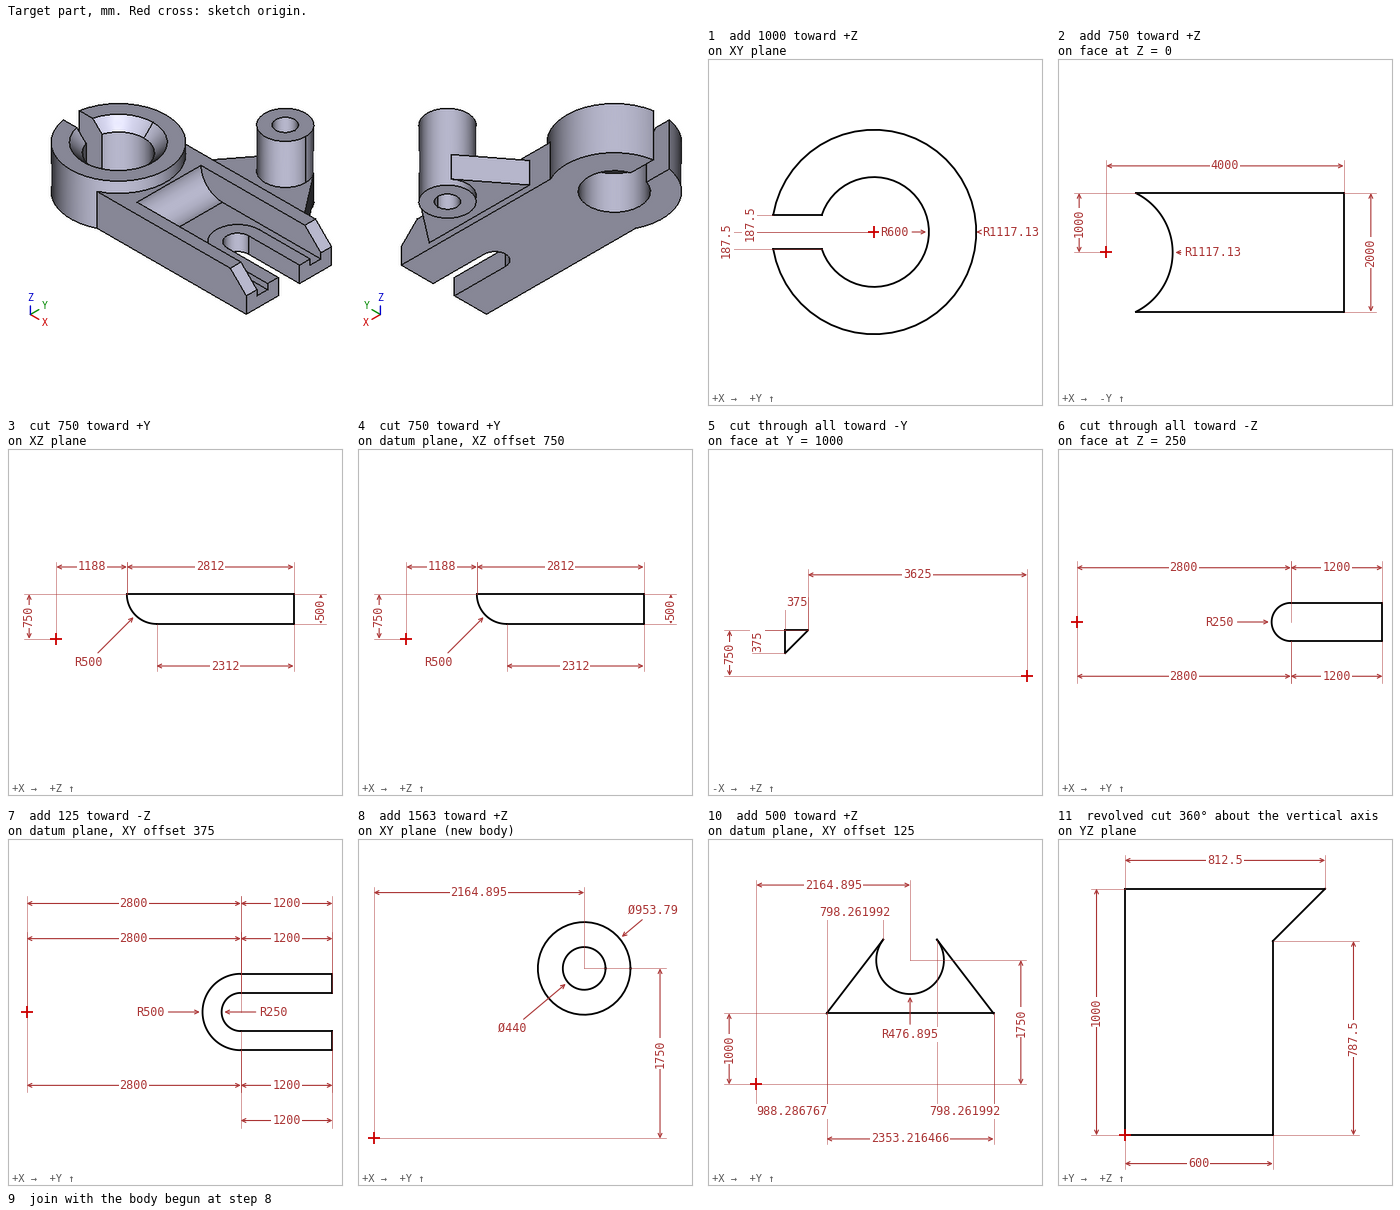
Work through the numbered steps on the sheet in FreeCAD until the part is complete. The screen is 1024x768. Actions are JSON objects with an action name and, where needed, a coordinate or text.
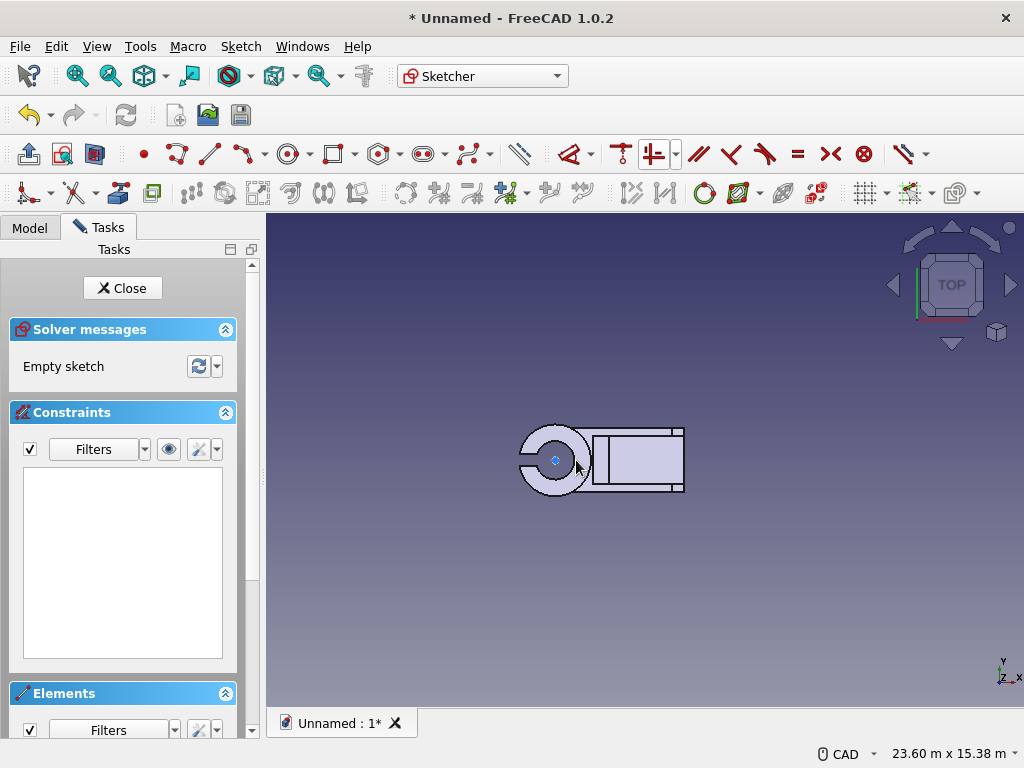
{"action": "scroll", "coordinate": [671, 460], "scroll_direction": "up", "scroll_amount": 11}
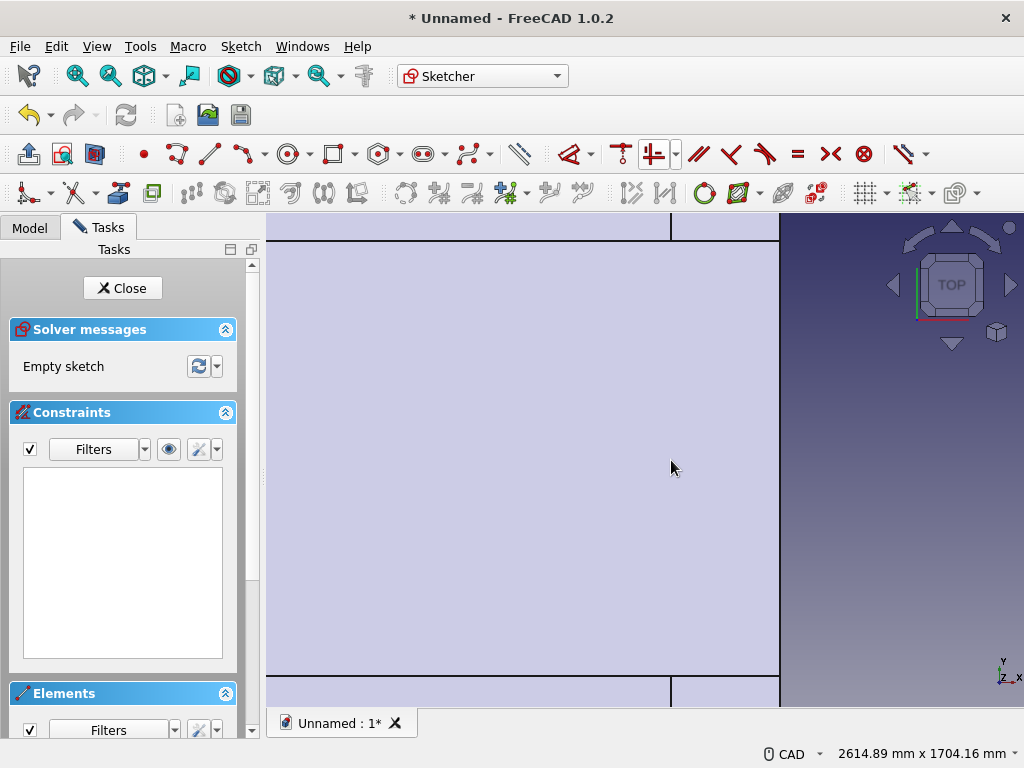
{"action": "key", "text": "g m"}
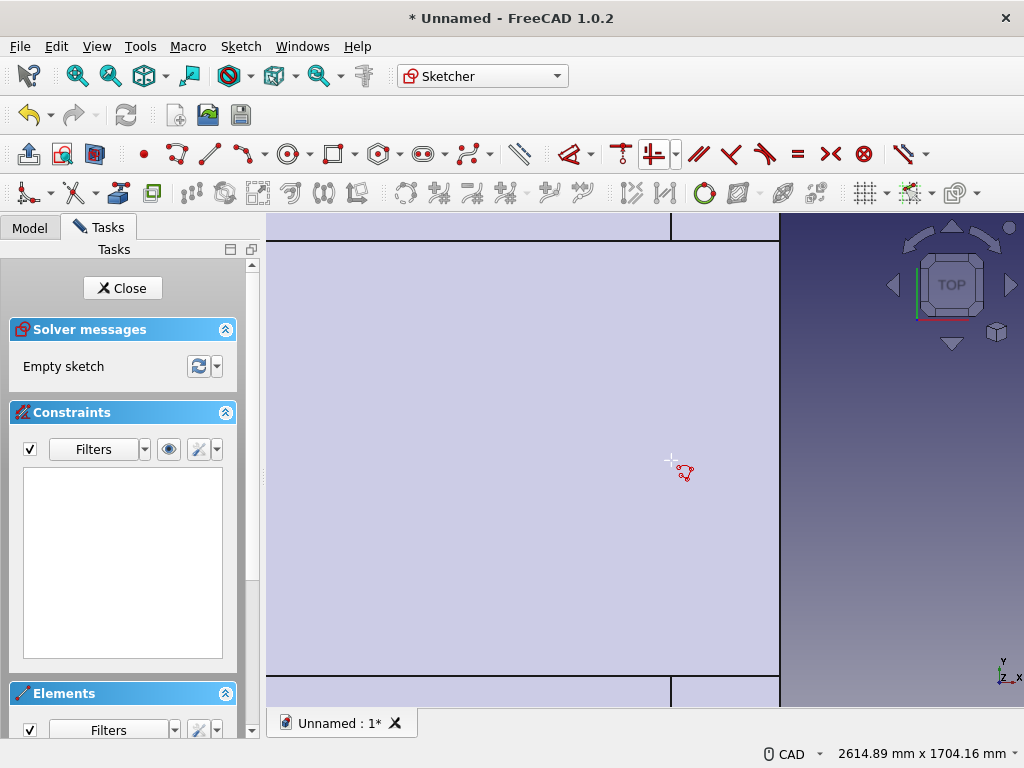
{"action": "left_click", "coordinate": [432, 531]}
{"action": "left_click", "coordinate": [780, 531]}
{"action": "left_click", "coordinate": [780, 386]}
{"action": "left_click", "coordinate": [432, 386]}
{"action": "right_click", "coordinate": [432, 386]}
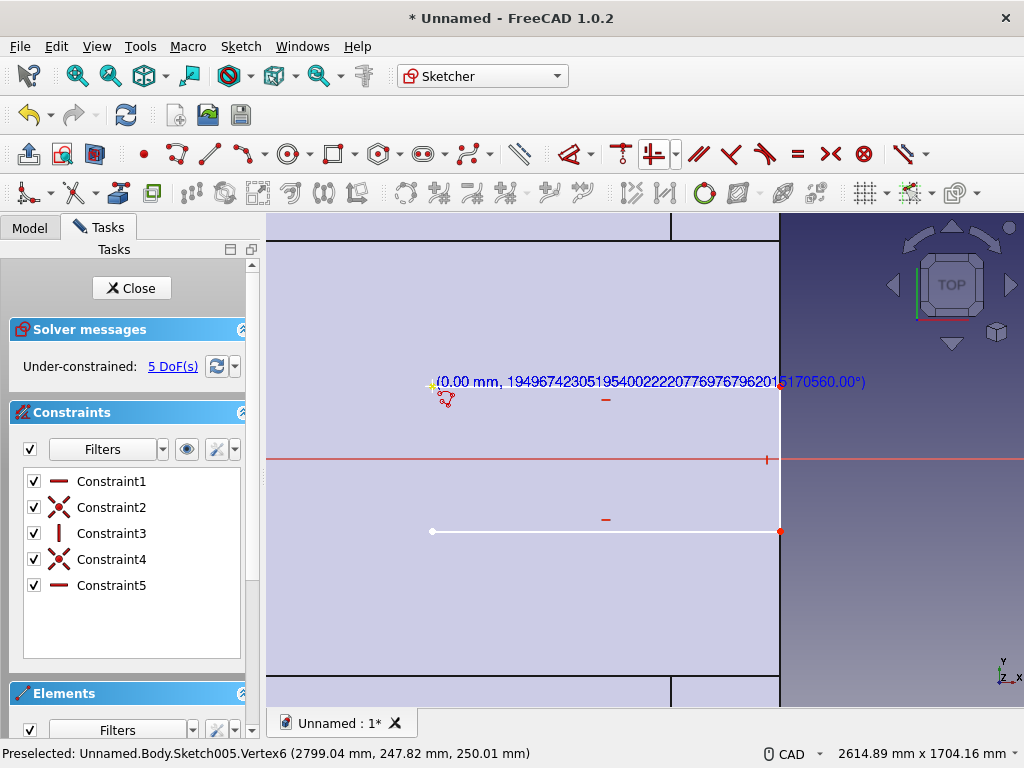
{"action": "key", "text": "g 3 a"}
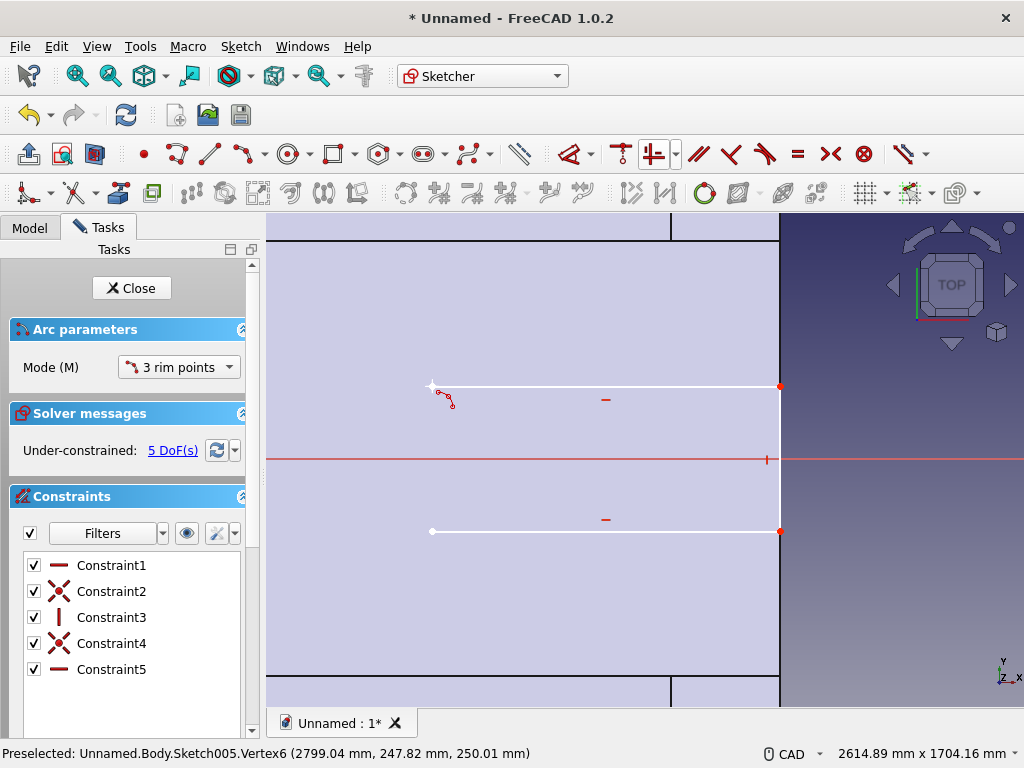
{"action": "left_click", "coordinate": [432, 387]}
{"action": "left_click", "coordinate": [432, 532]}
{"action": "left_click", "coordinate": [363, 436]}
{"action": "key", "text": "Escape"}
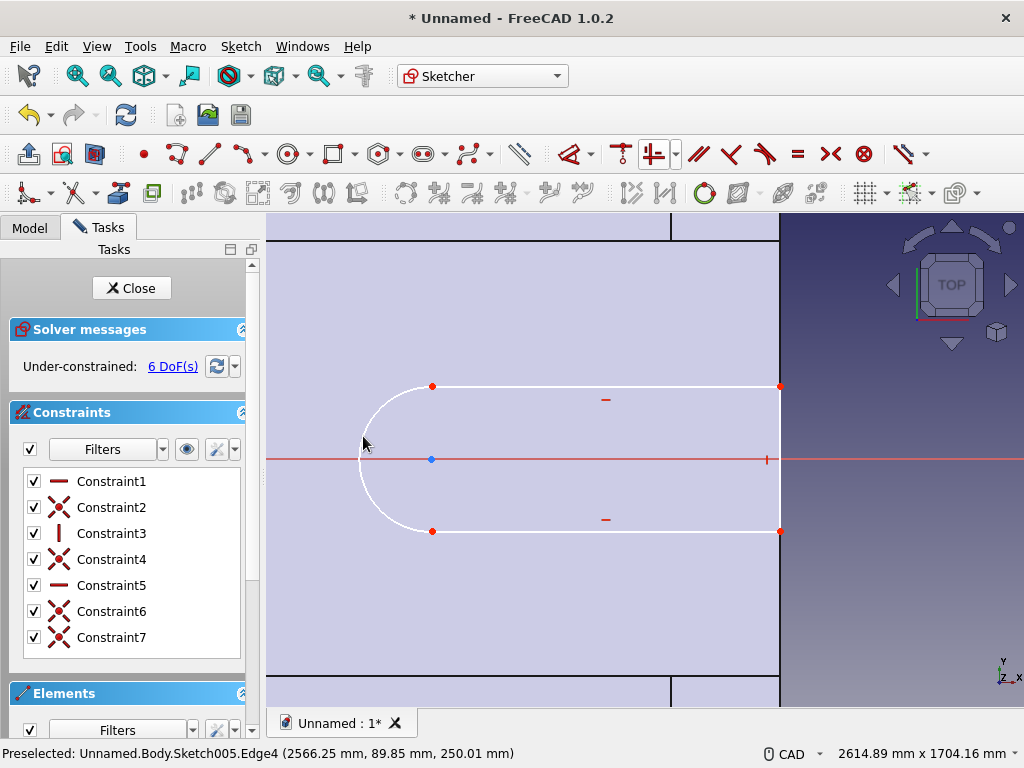
{"action": "left_click", "coordinate": [432, 460]}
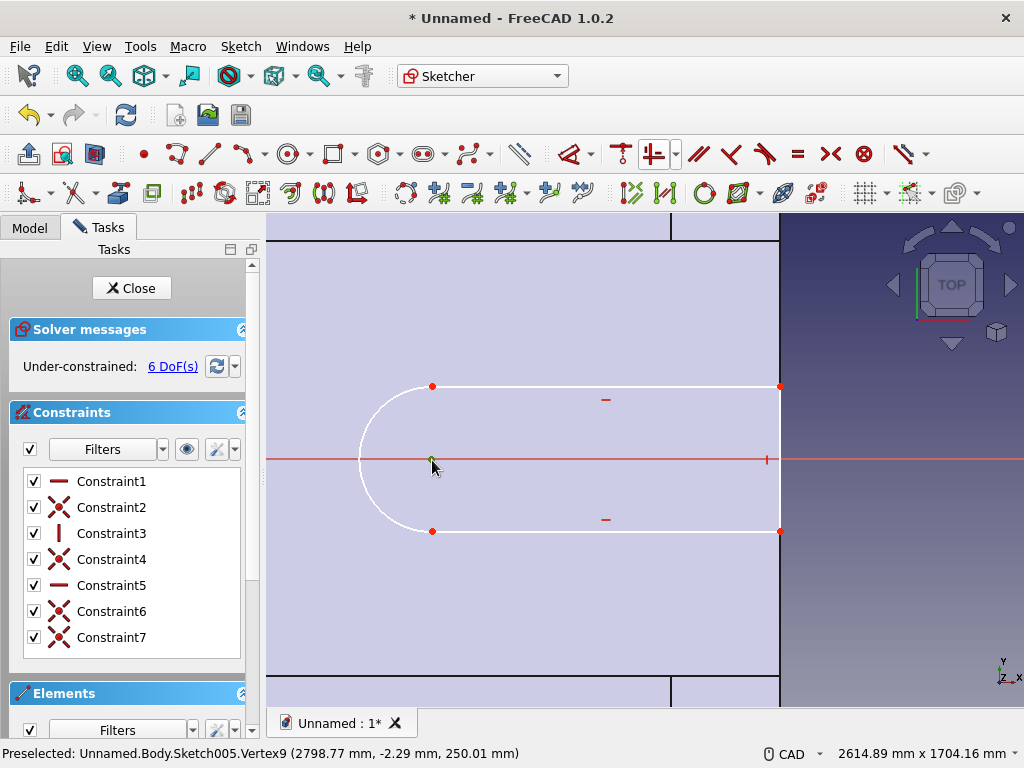
{"action": "left_click", "coordinate": [415, 459]}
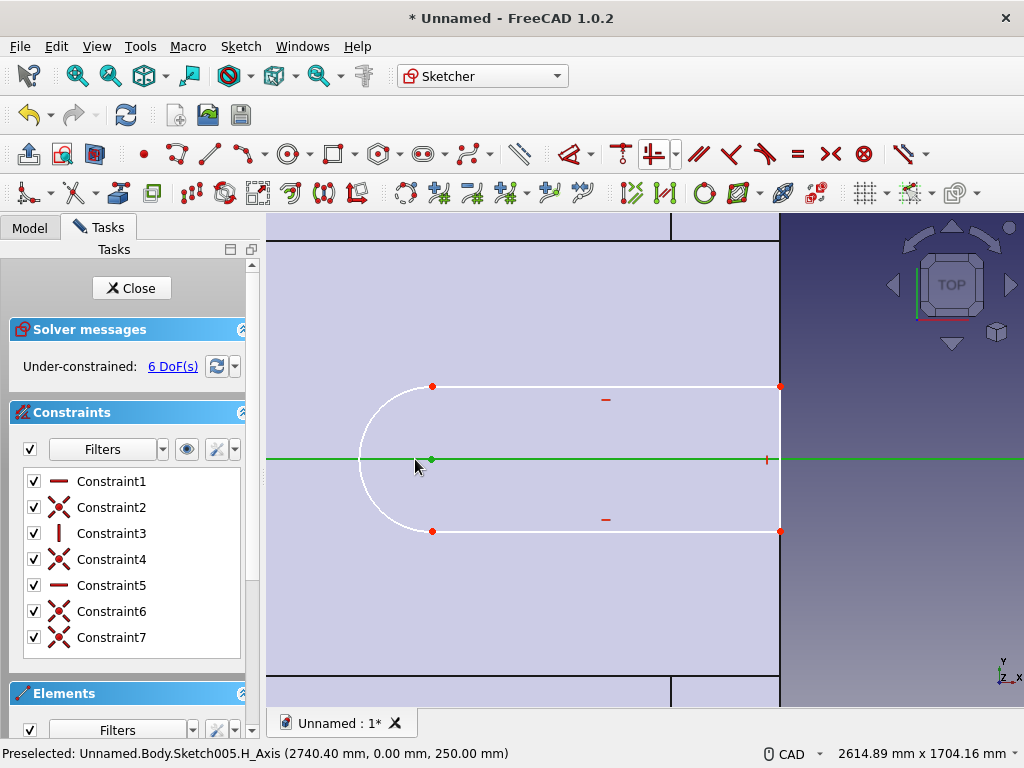
{"action": "key", "text": "c"}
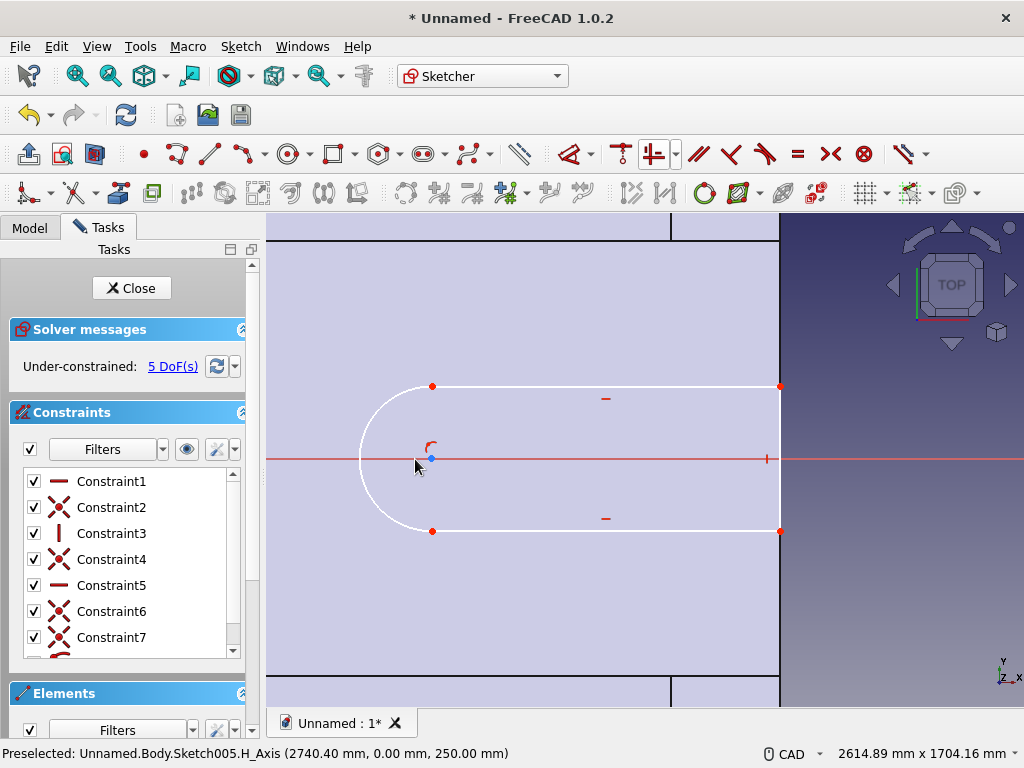
{"action": "key", "text": "d"}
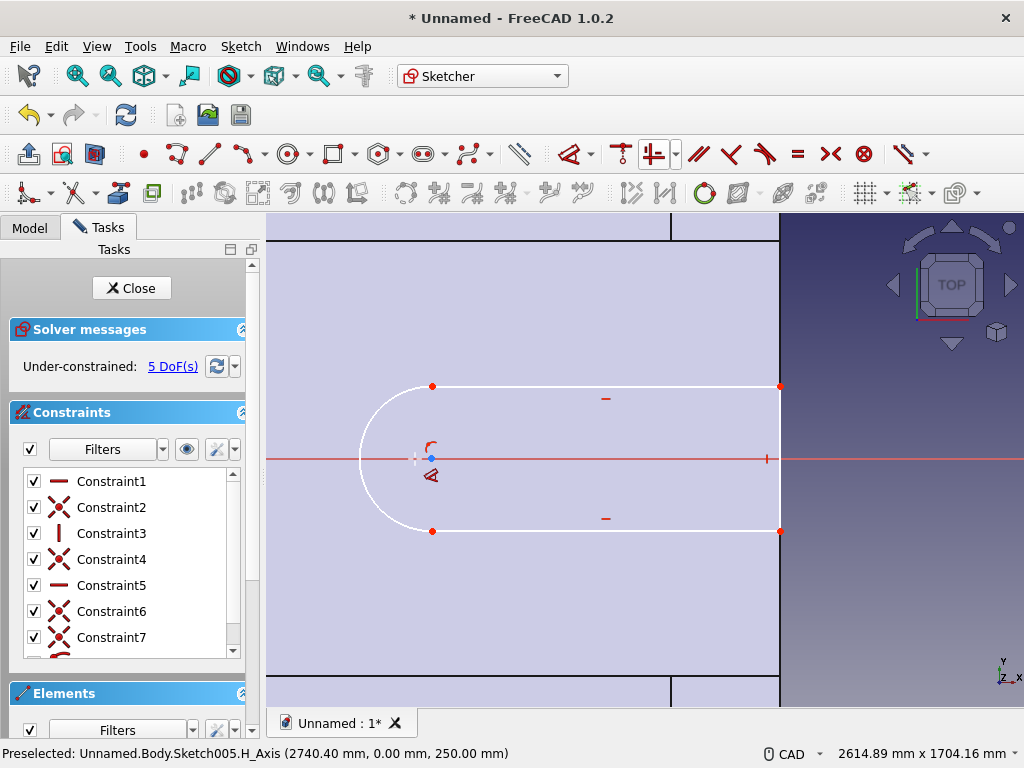
{"action": "left_click", "coordinate": [373, 416]}
{"action": "left_click", "coordinate": [347, 397]}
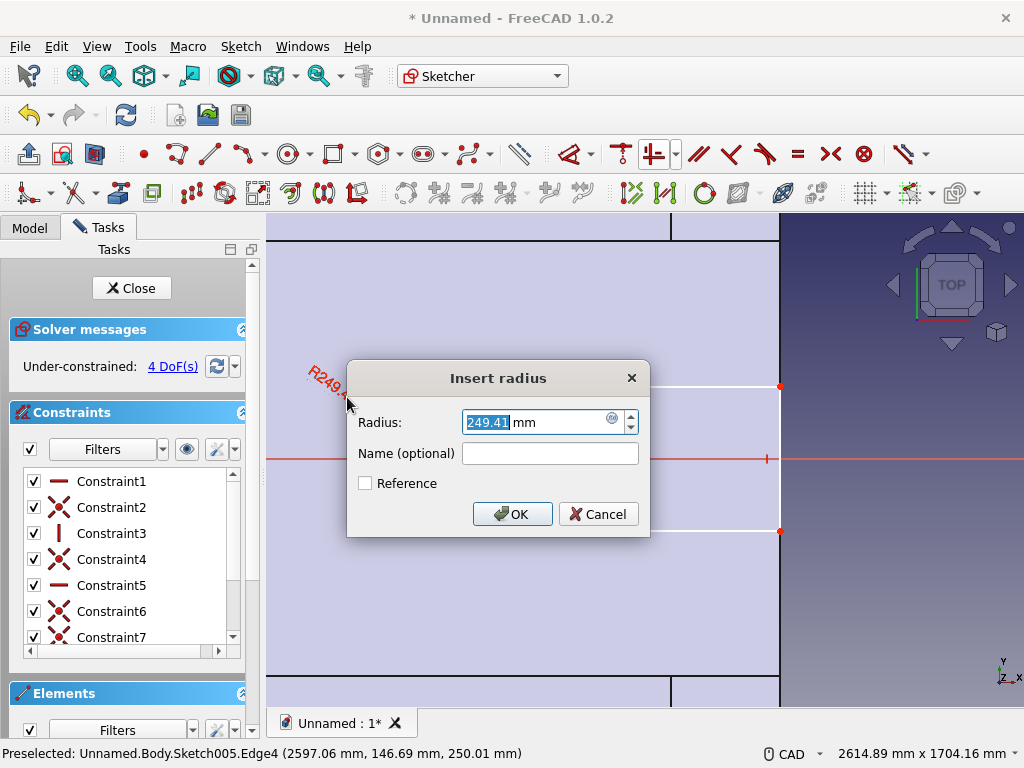
{"action": "type", "text": "250"}
{"action": "key", "text": "Return"}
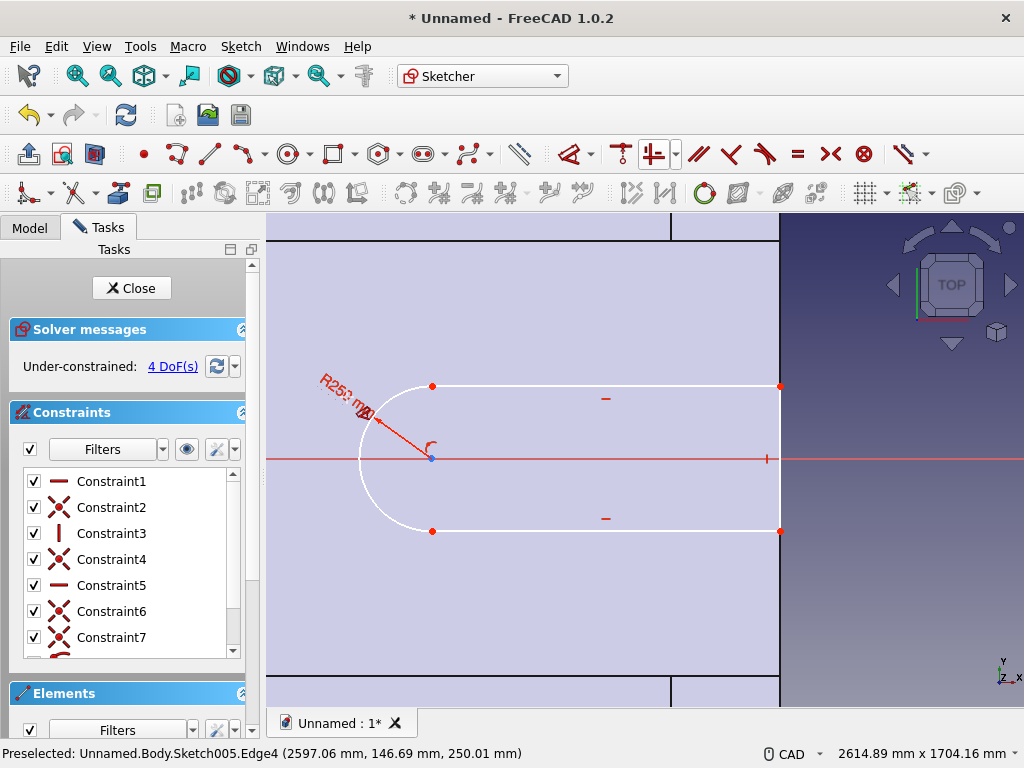
{"action": "left_click", "coordinate": [536, 531]}
{"action": "left_click", "coordinate": [606, 565]}